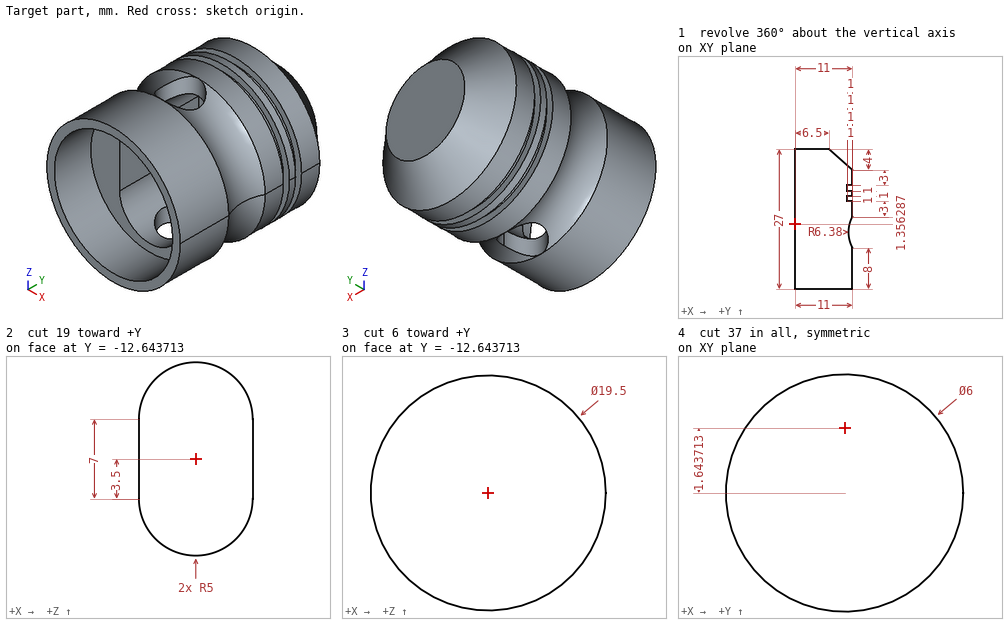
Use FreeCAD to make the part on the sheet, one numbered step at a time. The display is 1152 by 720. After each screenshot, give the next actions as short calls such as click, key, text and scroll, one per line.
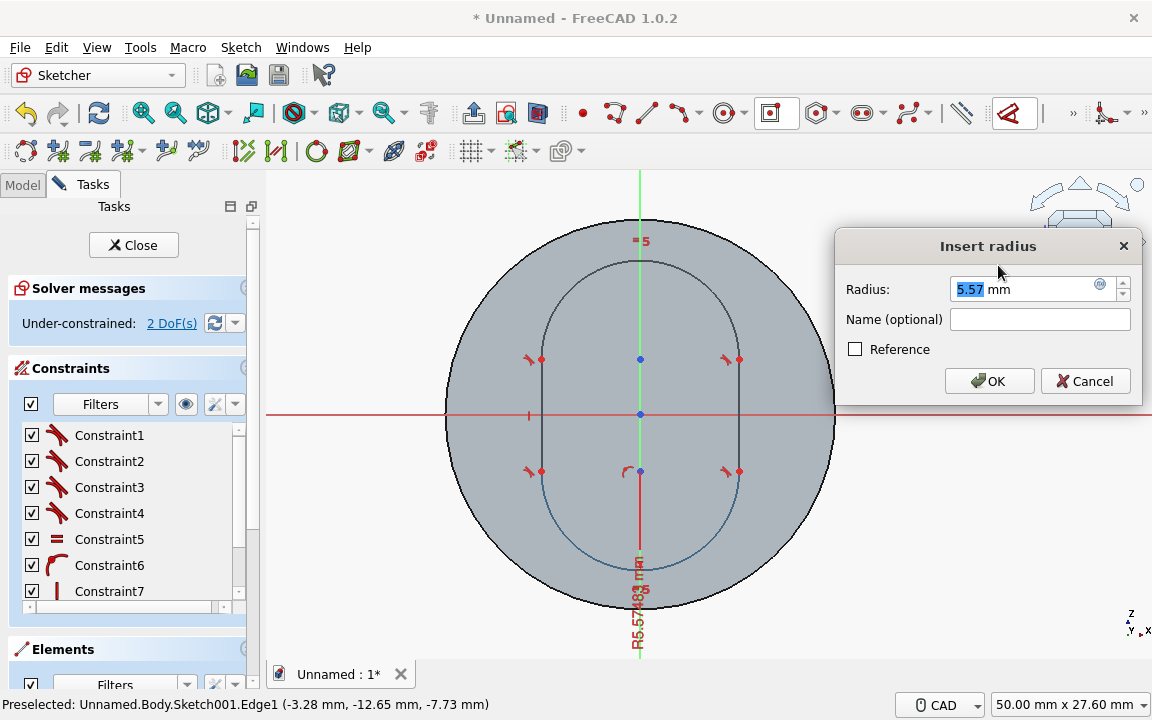
text(5)
key(Return)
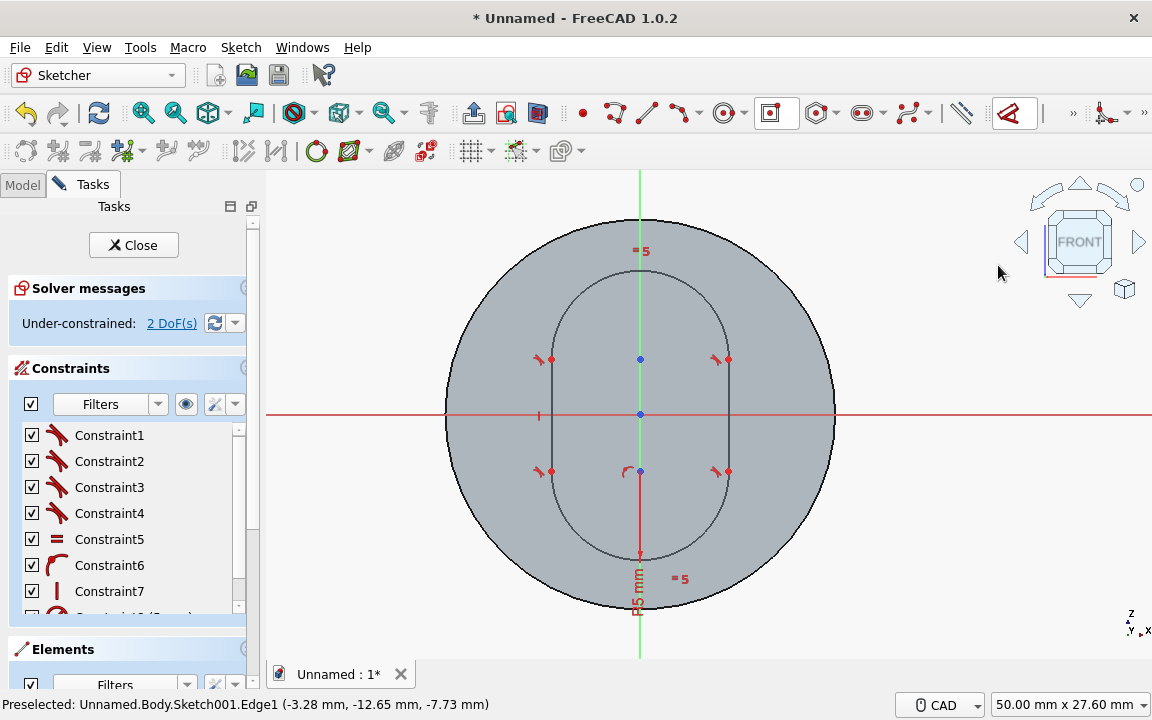
click(552, 438)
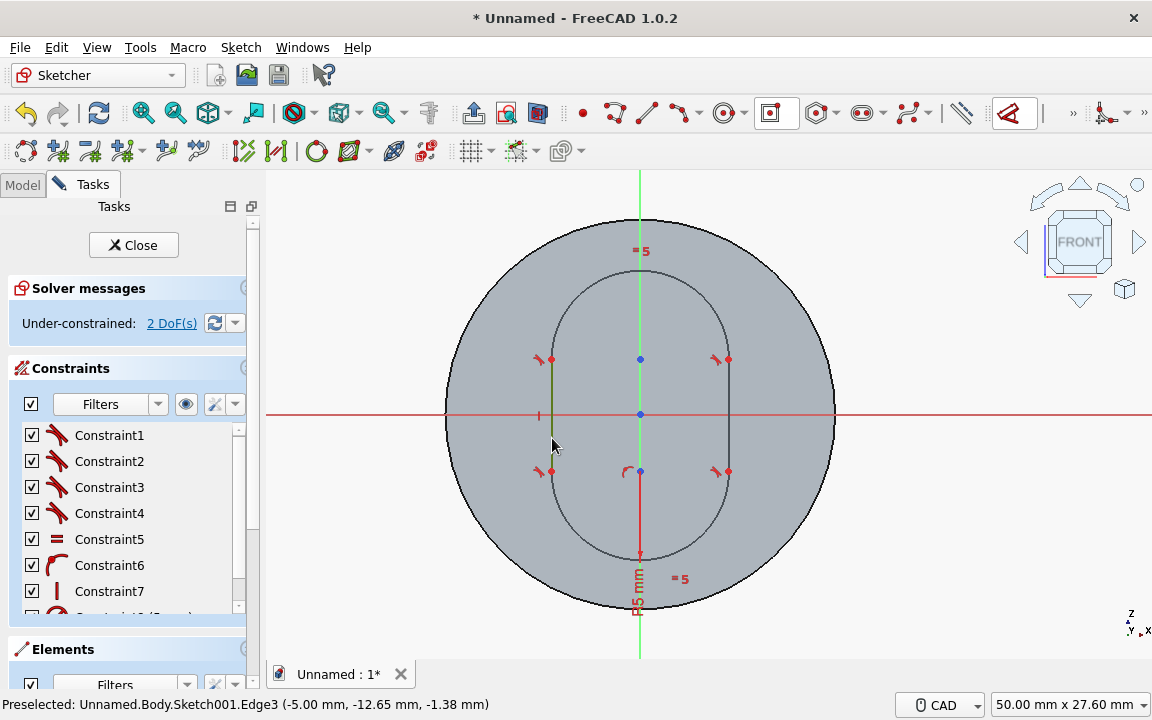
click(1032, 114)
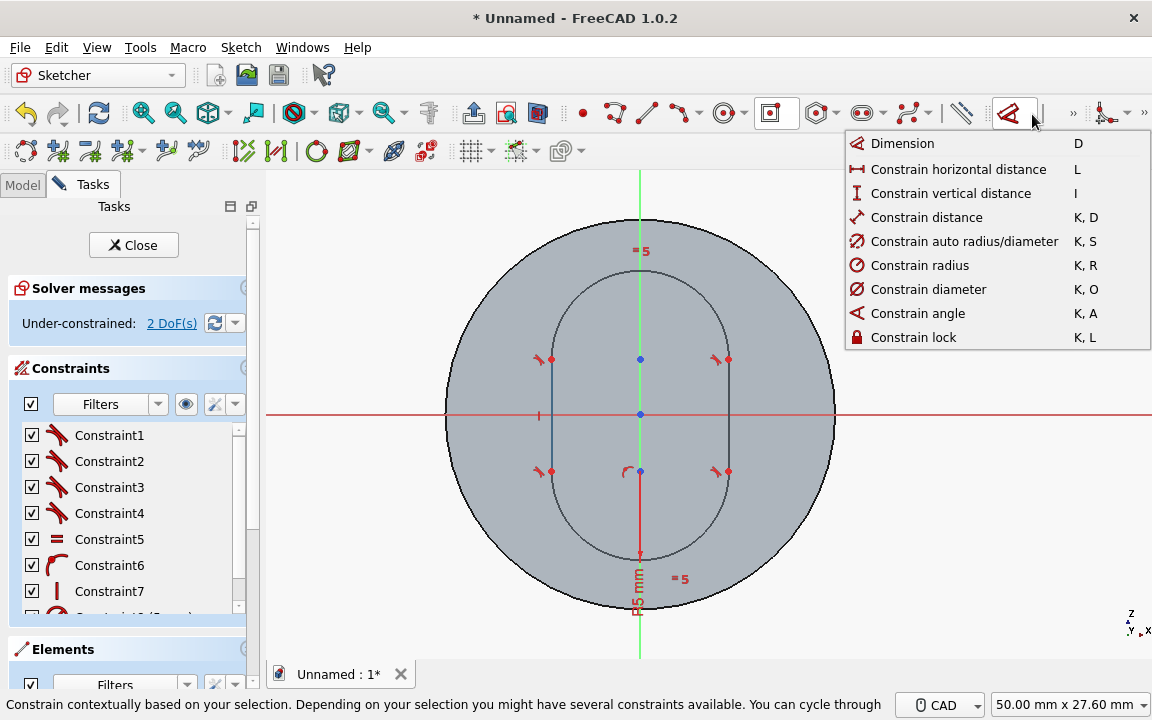
click(998, 193)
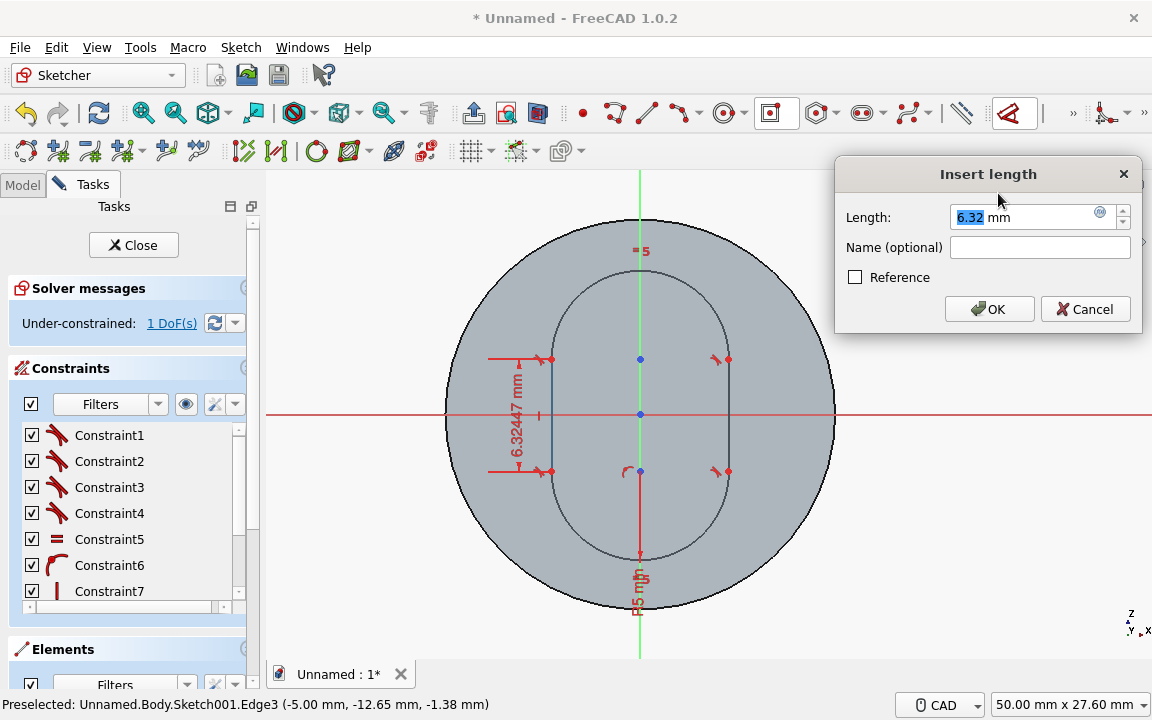
text(7)
key(Return)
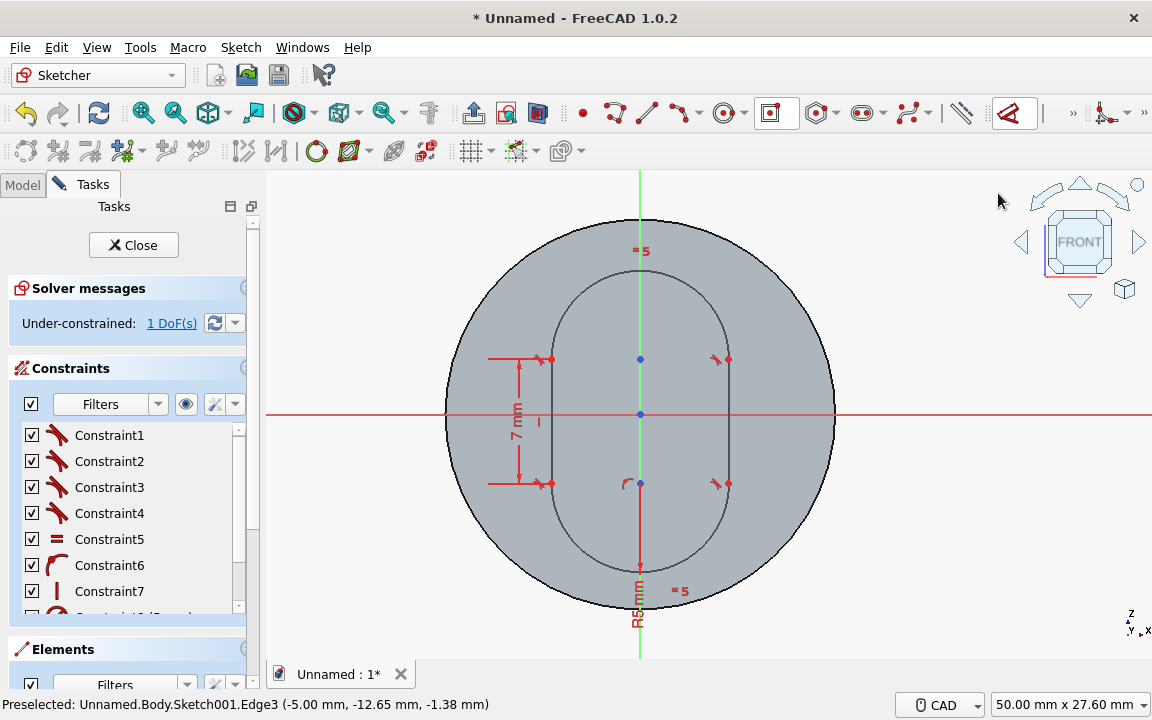
click(552, 484)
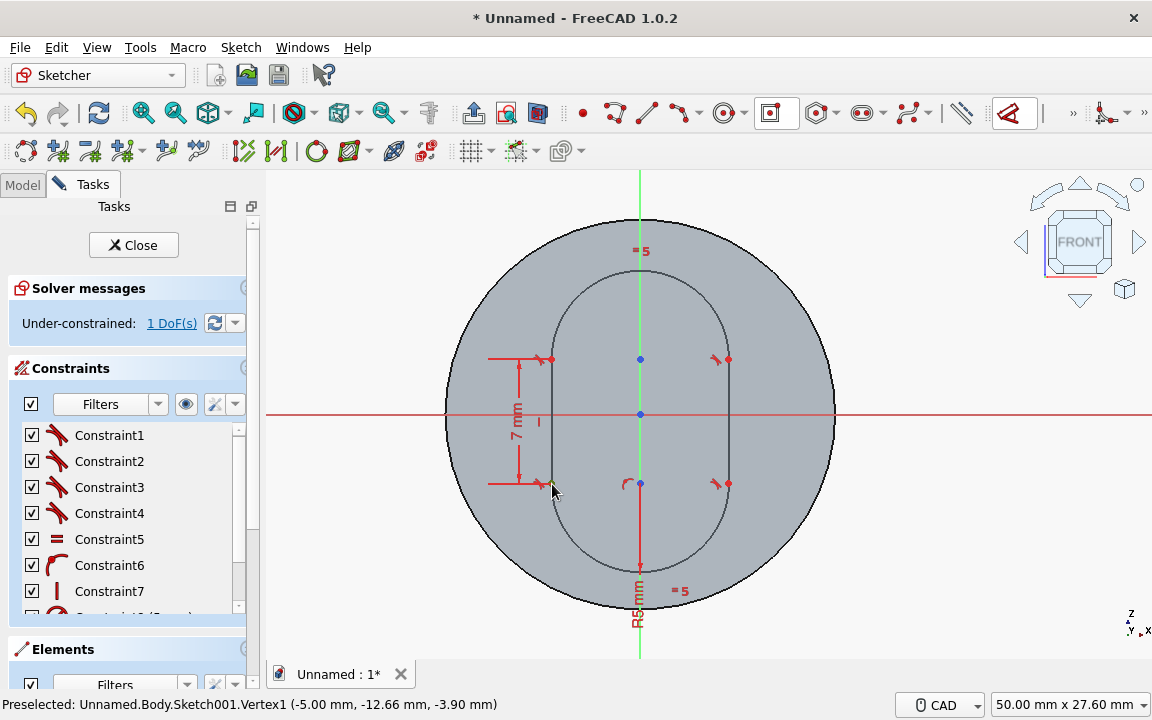
key(i)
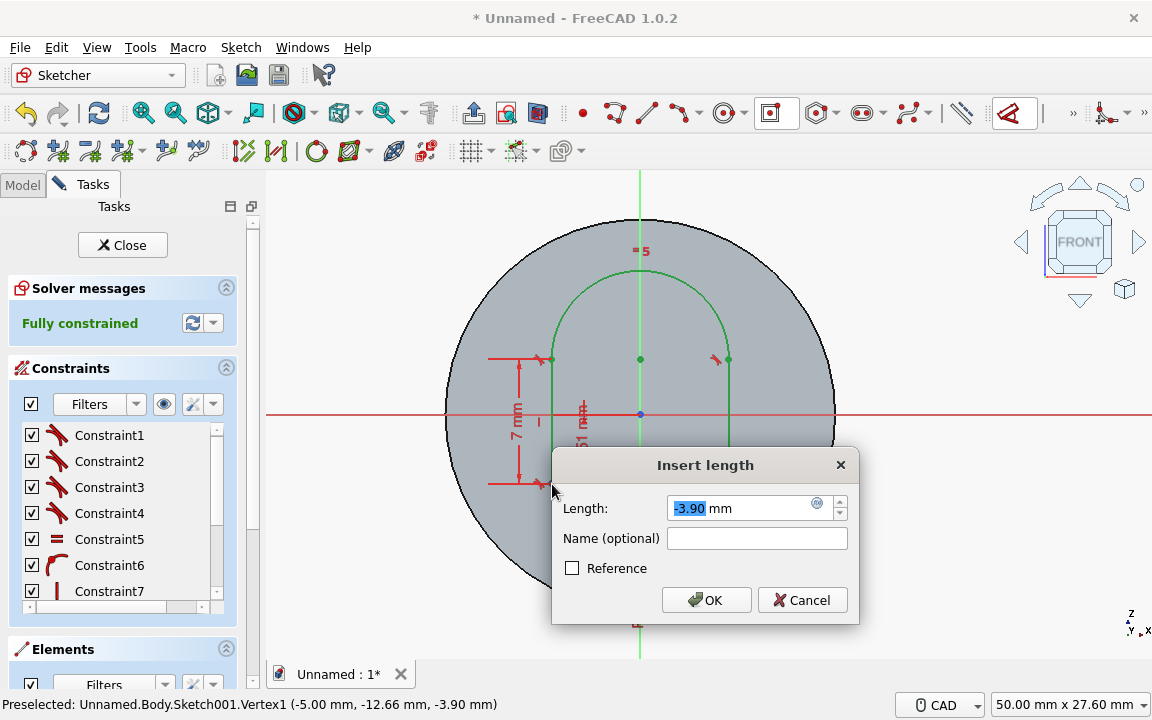
text(-3.5)
key(Return)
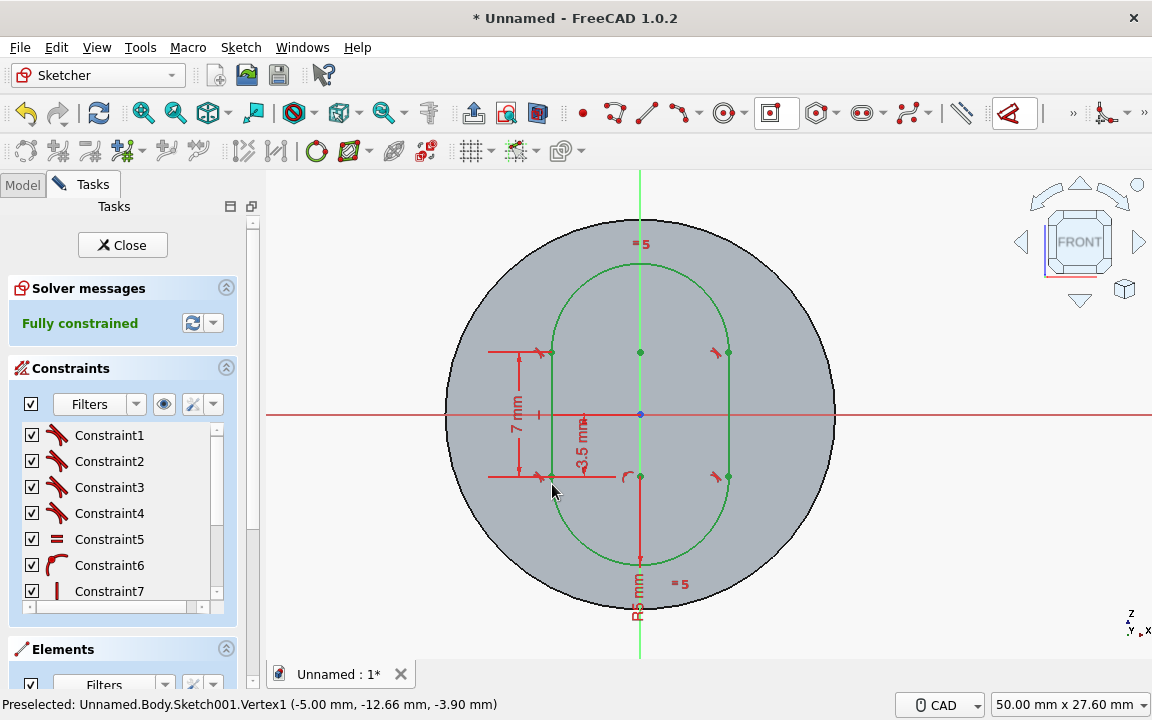
click(123, 245)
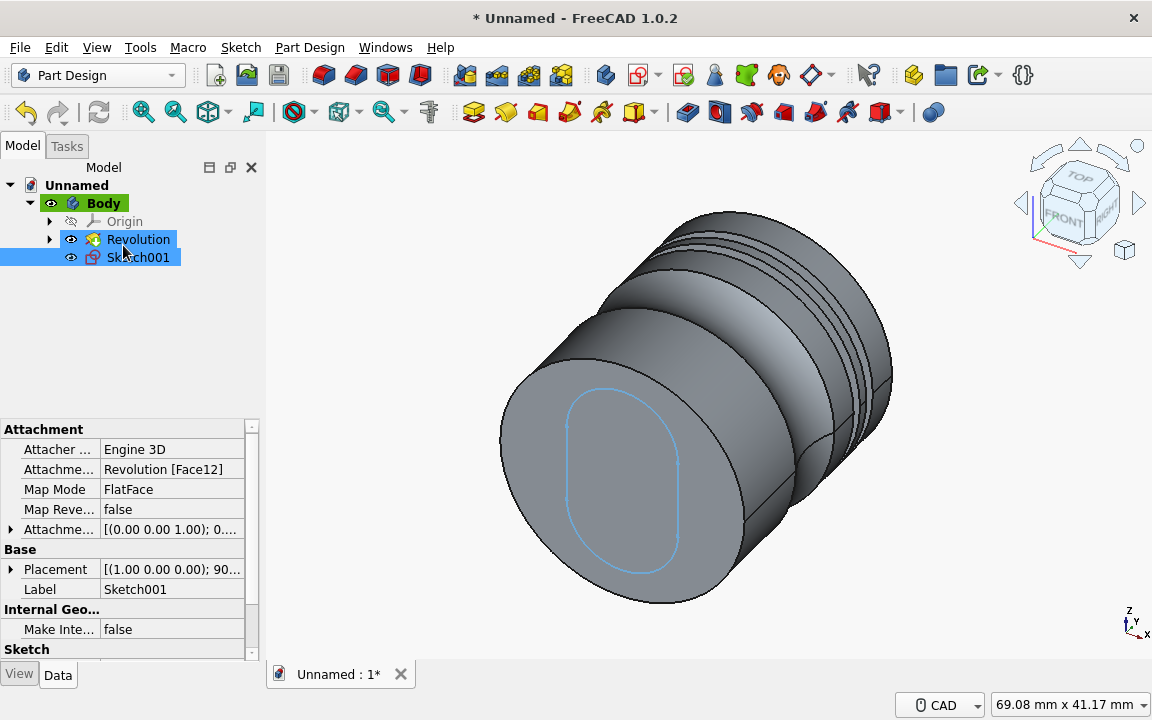
click(688, 112)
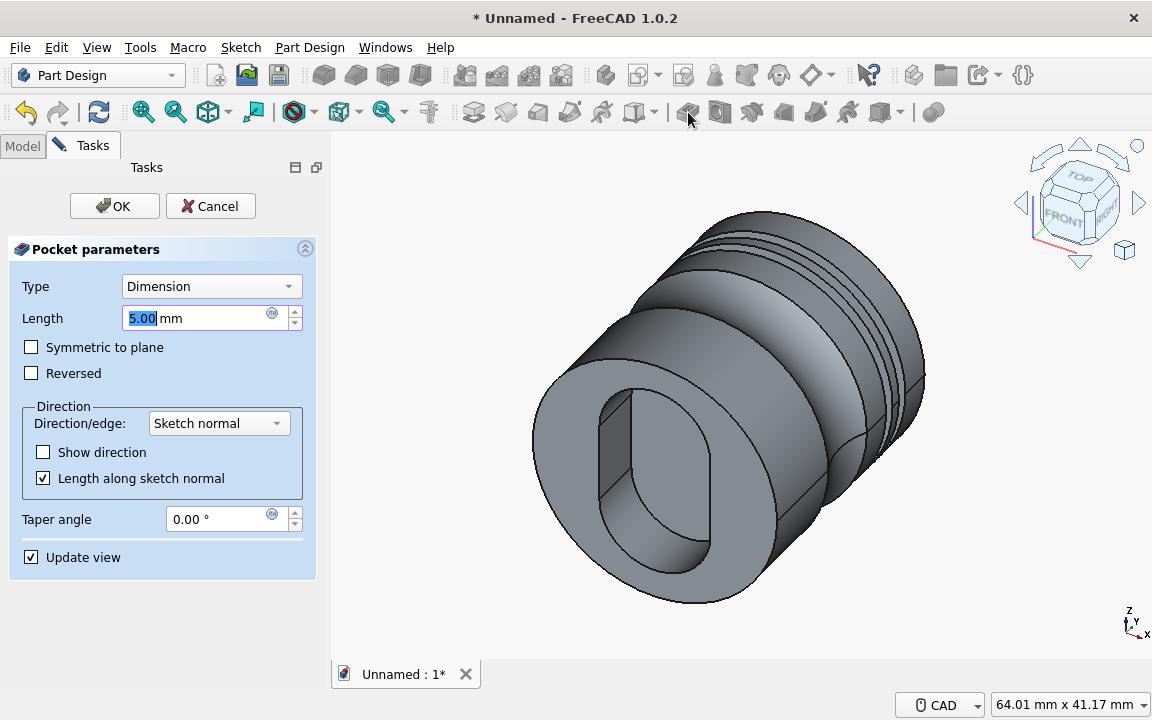
text(19)
key(Tab)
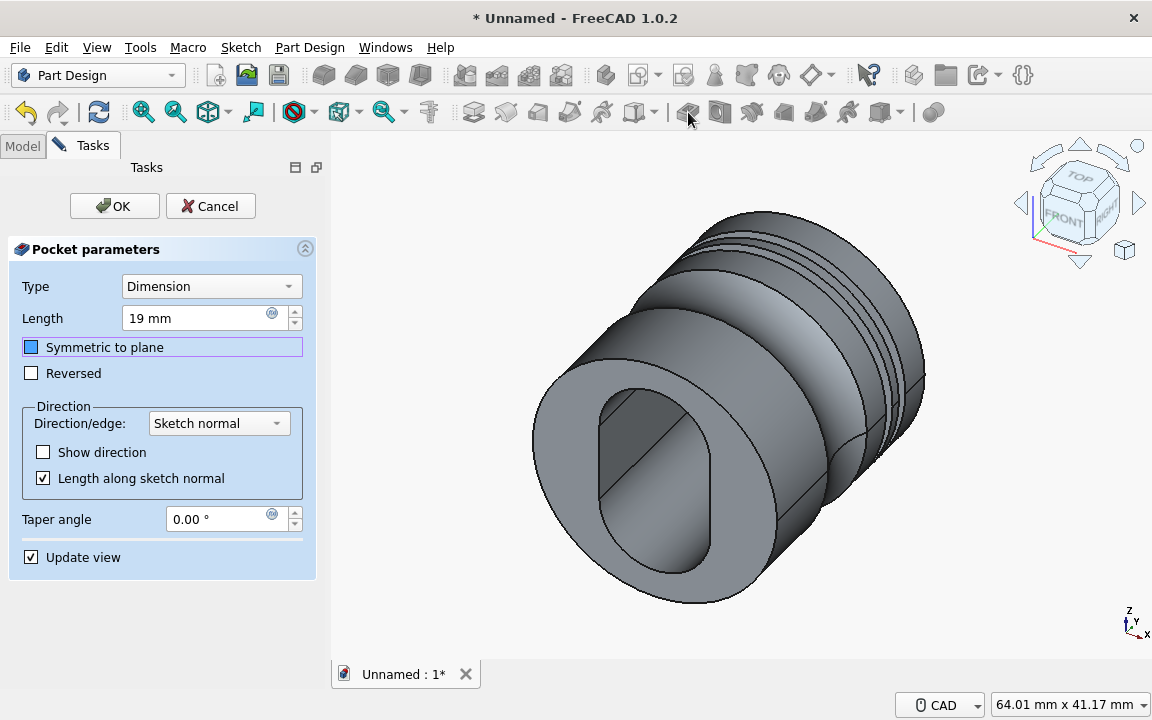
click(115, 206)